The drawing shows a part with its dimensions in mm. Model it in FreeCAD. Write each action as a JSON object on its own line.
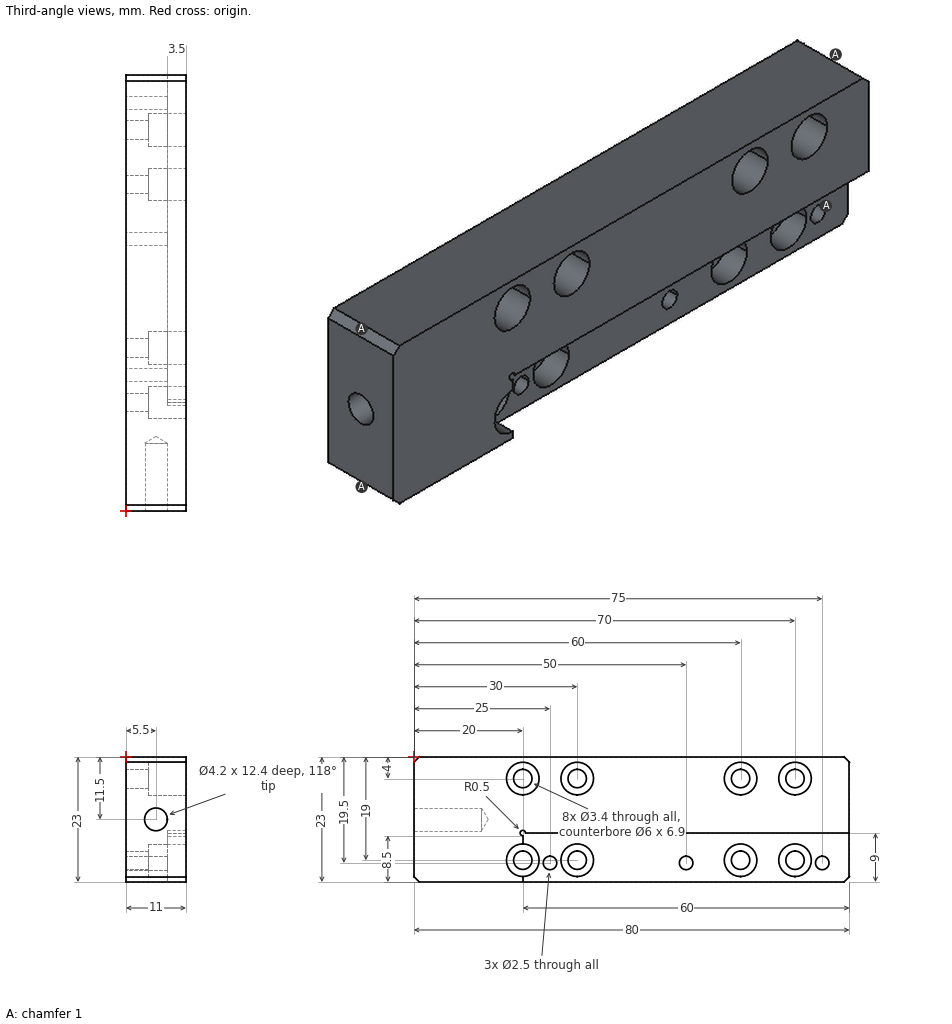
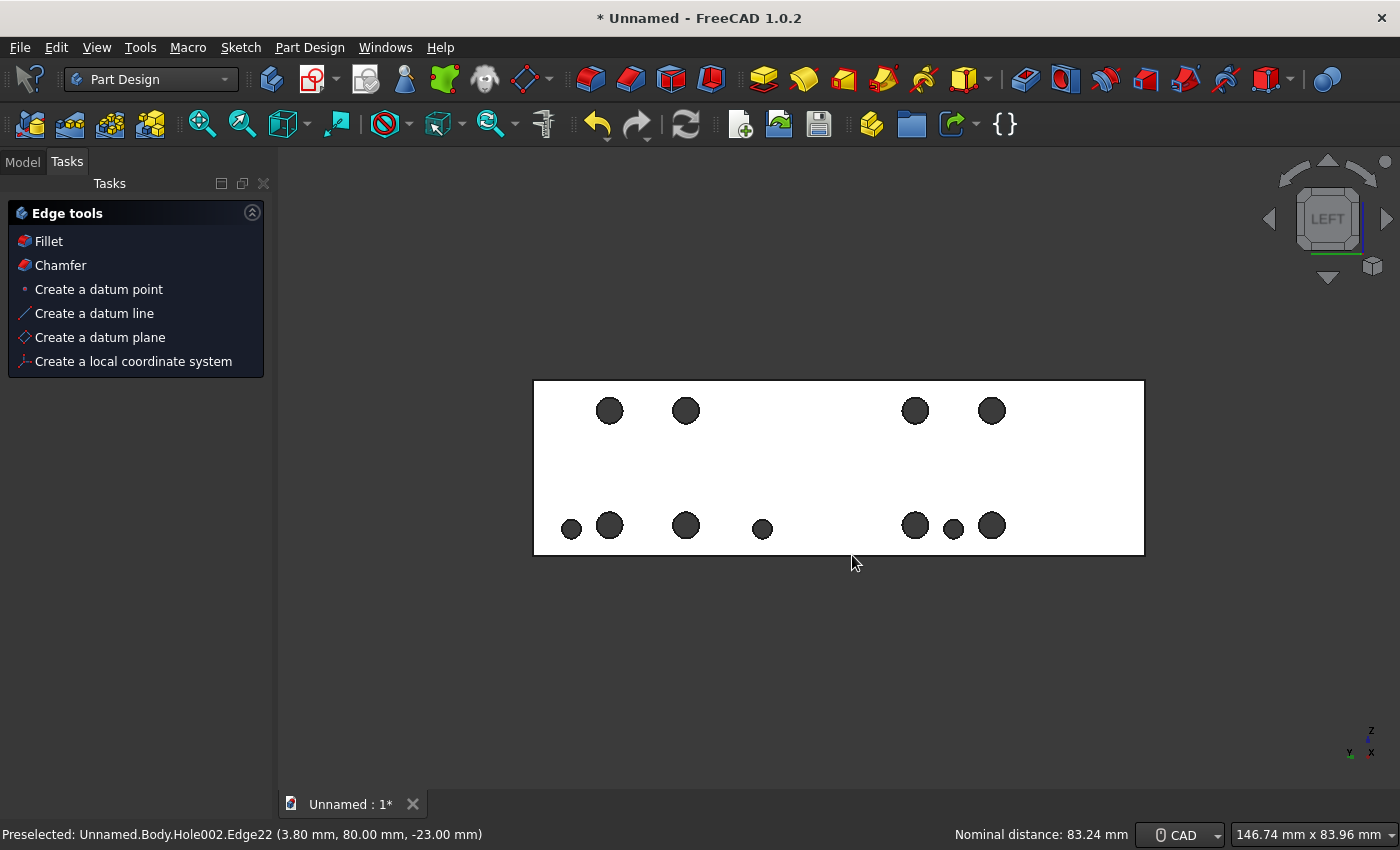
{"action": "key", "text": "v 3"}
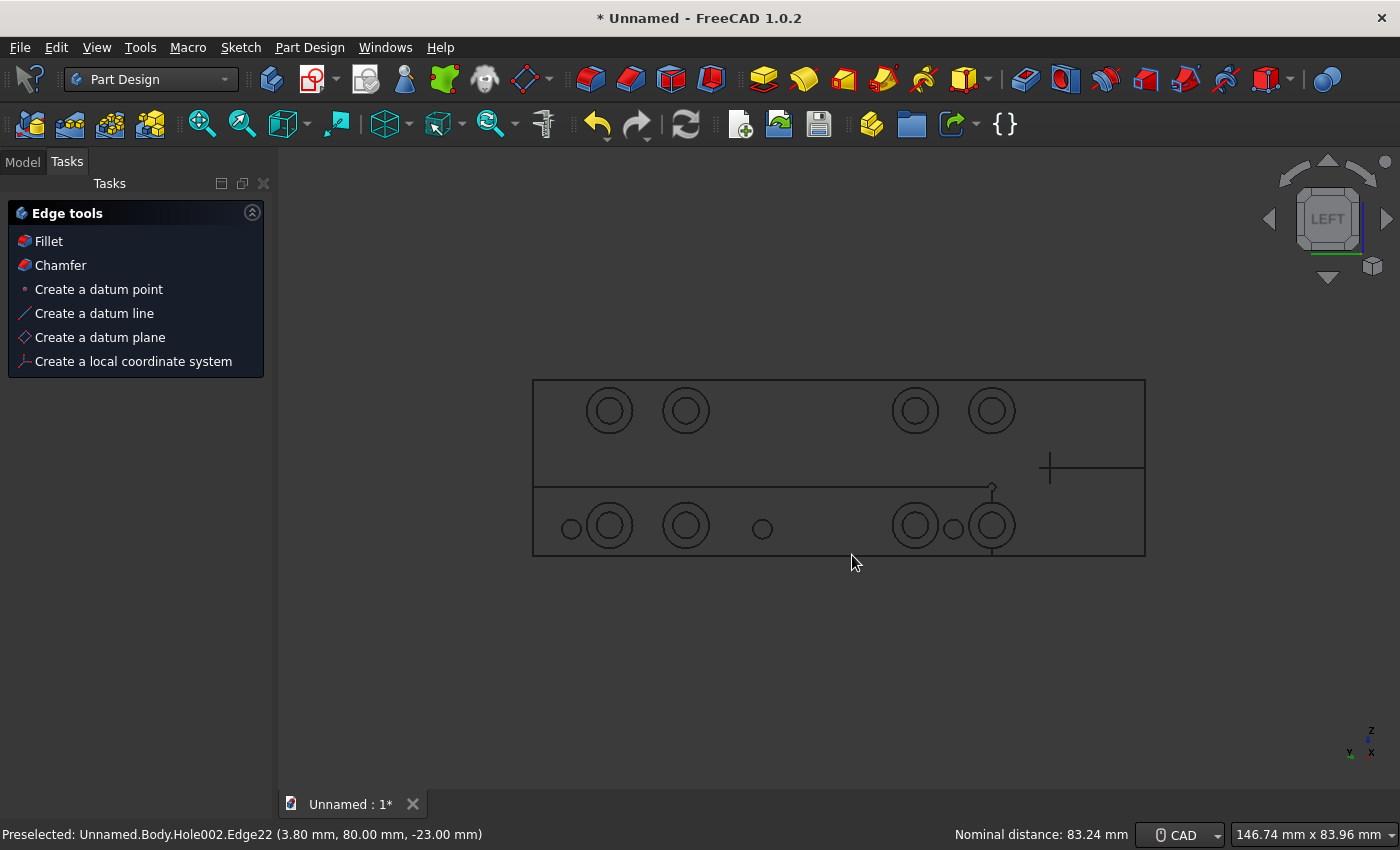
{"action": "key", "text": "0"}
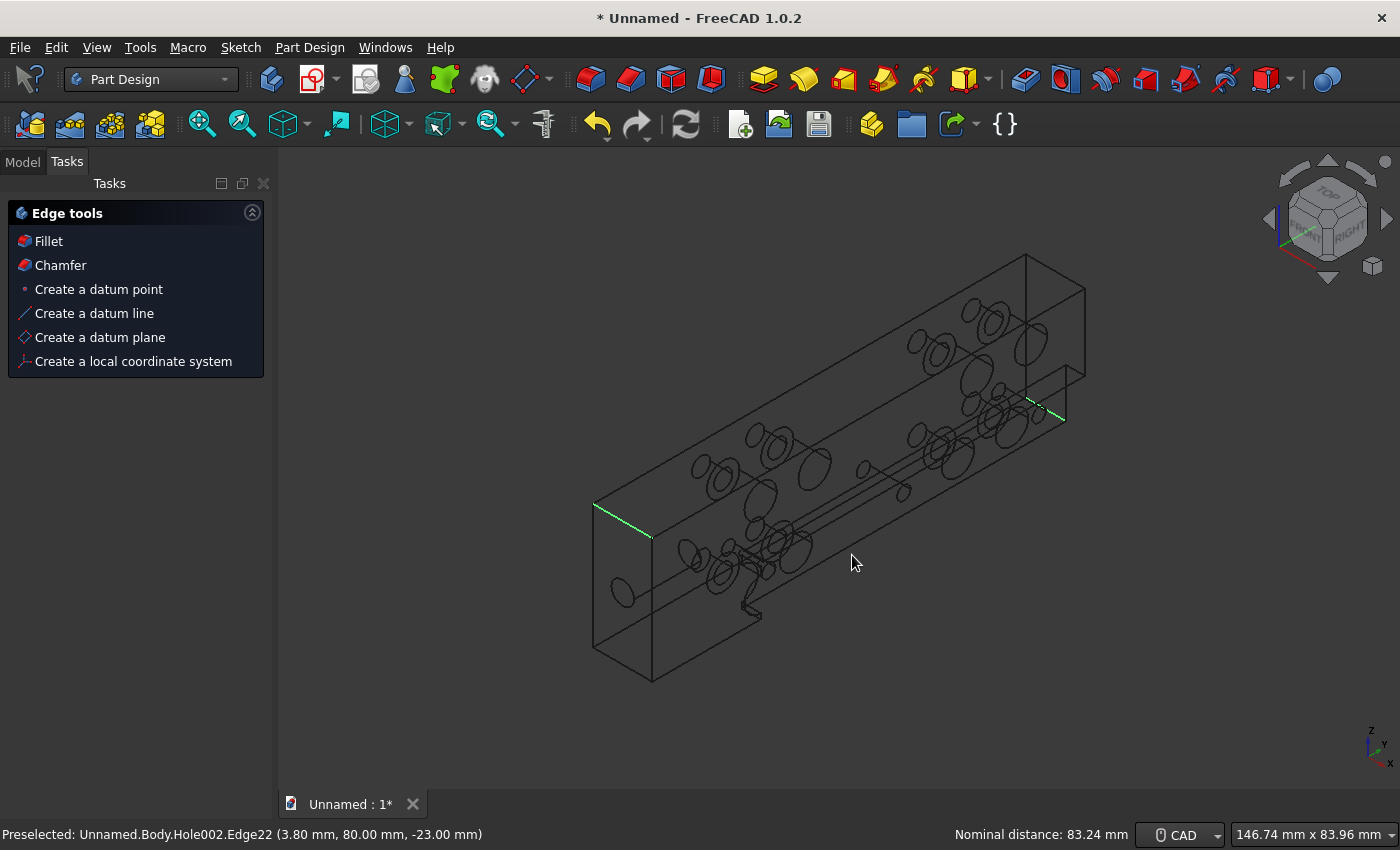
{"action": "left_click", "coordinate": [1055, 270], "text": "ctrl"}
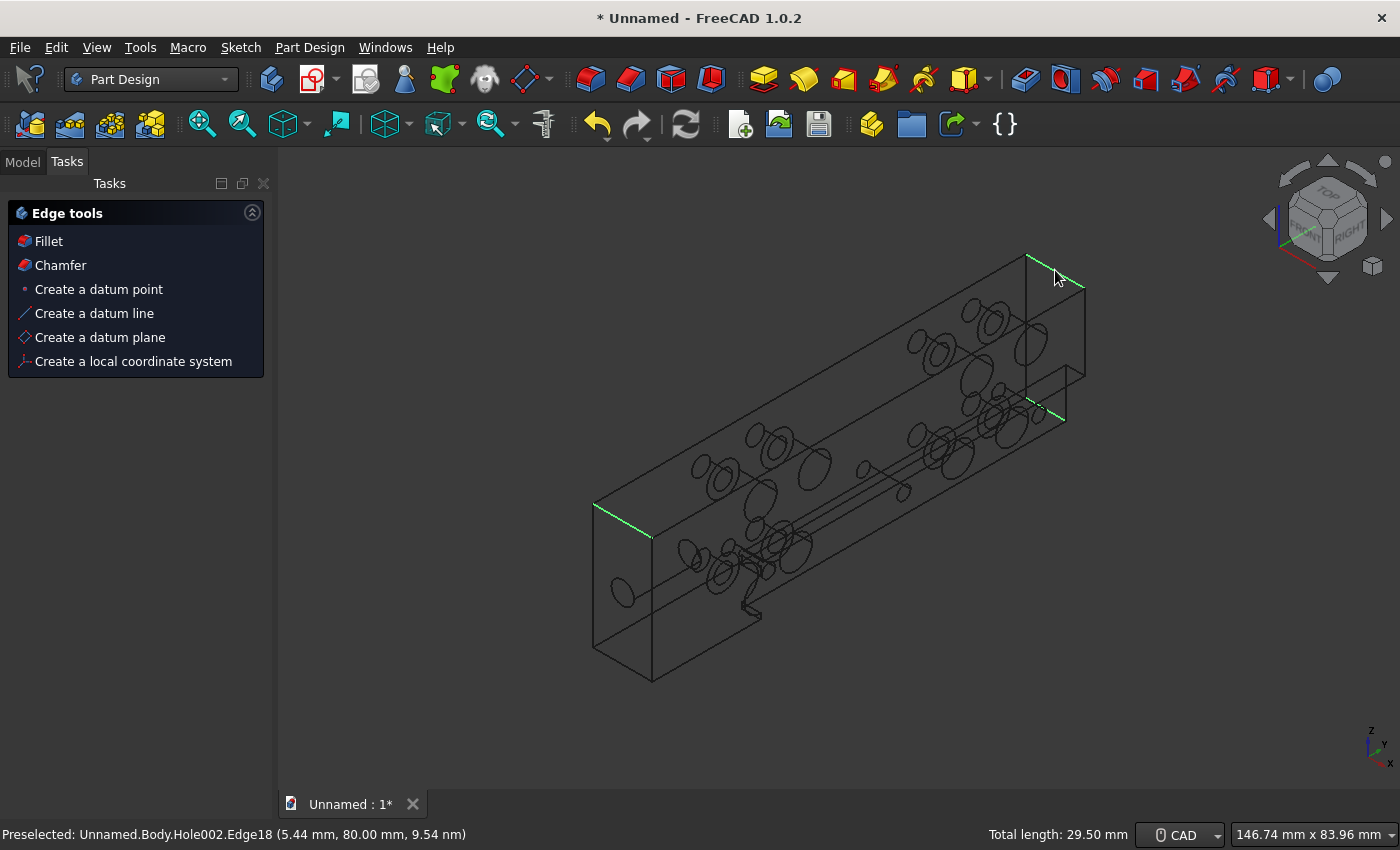
{"action": "left_click", "coordinate": [623, 664], "text": "ctrl"}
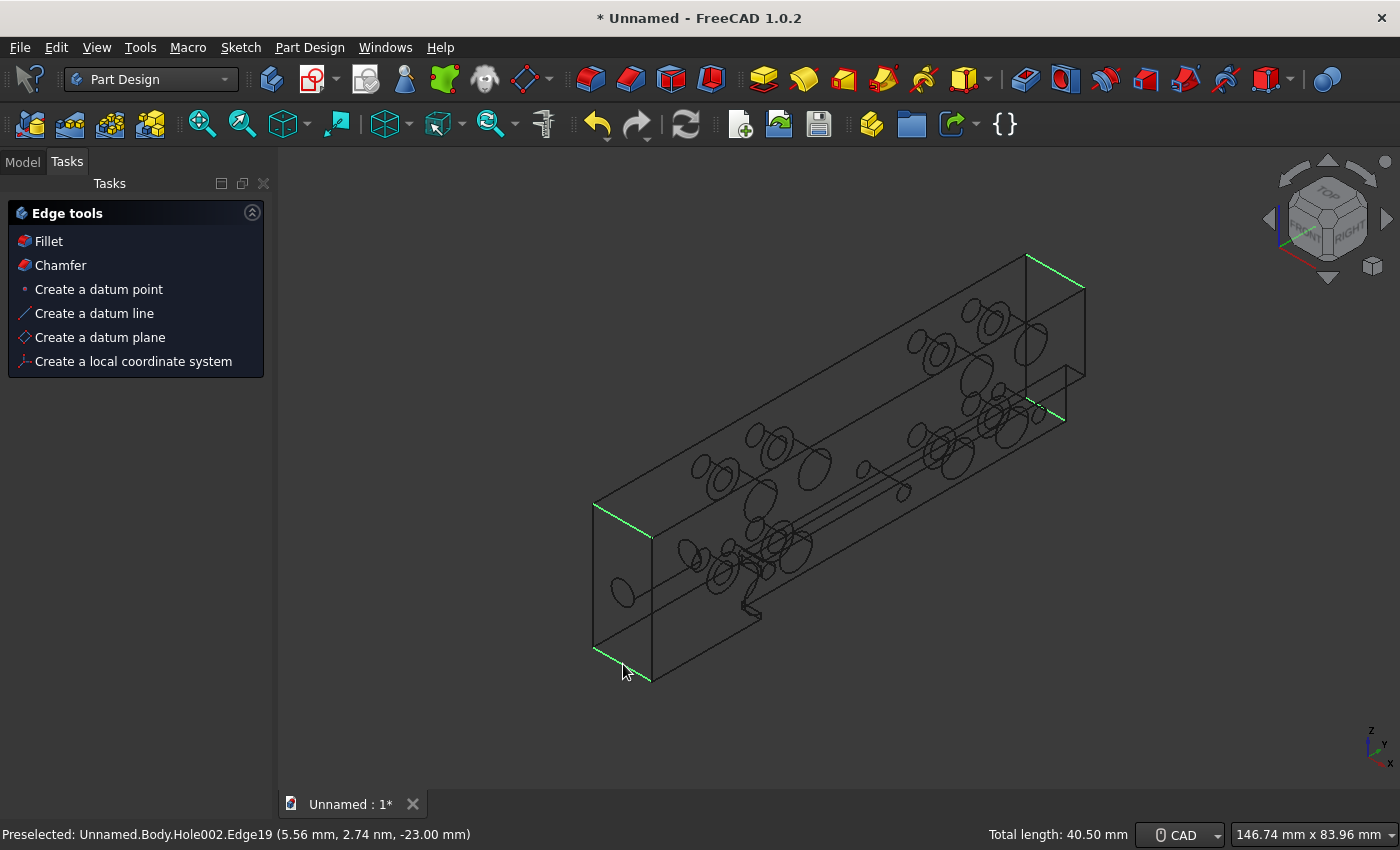
{"action": "key", "text": "v 1"}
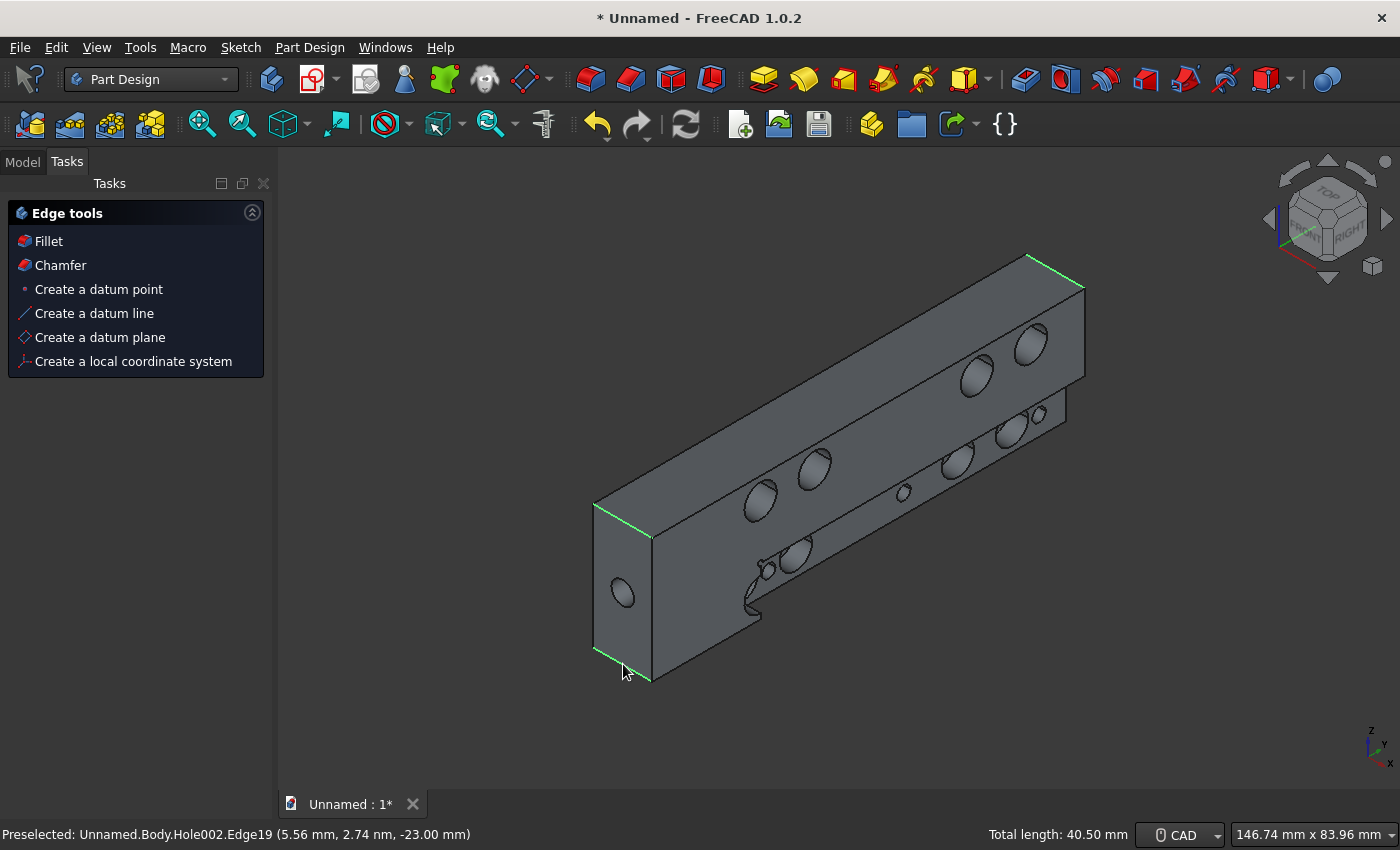
{"action": "left_click", "coordinate": [632, 80]}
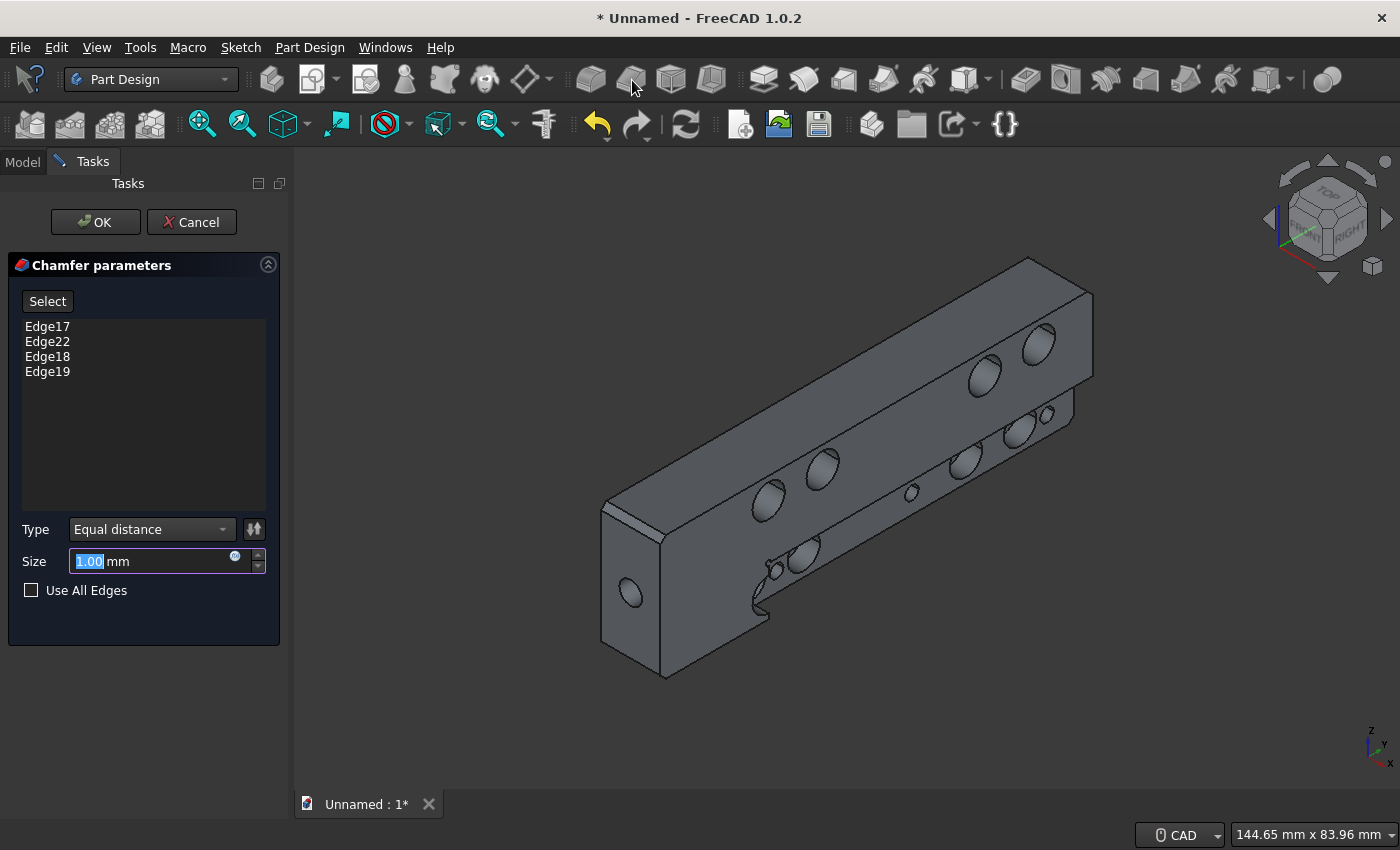
{"action": "type", "text": "1"}
{"action": "key", "text": "Tab"}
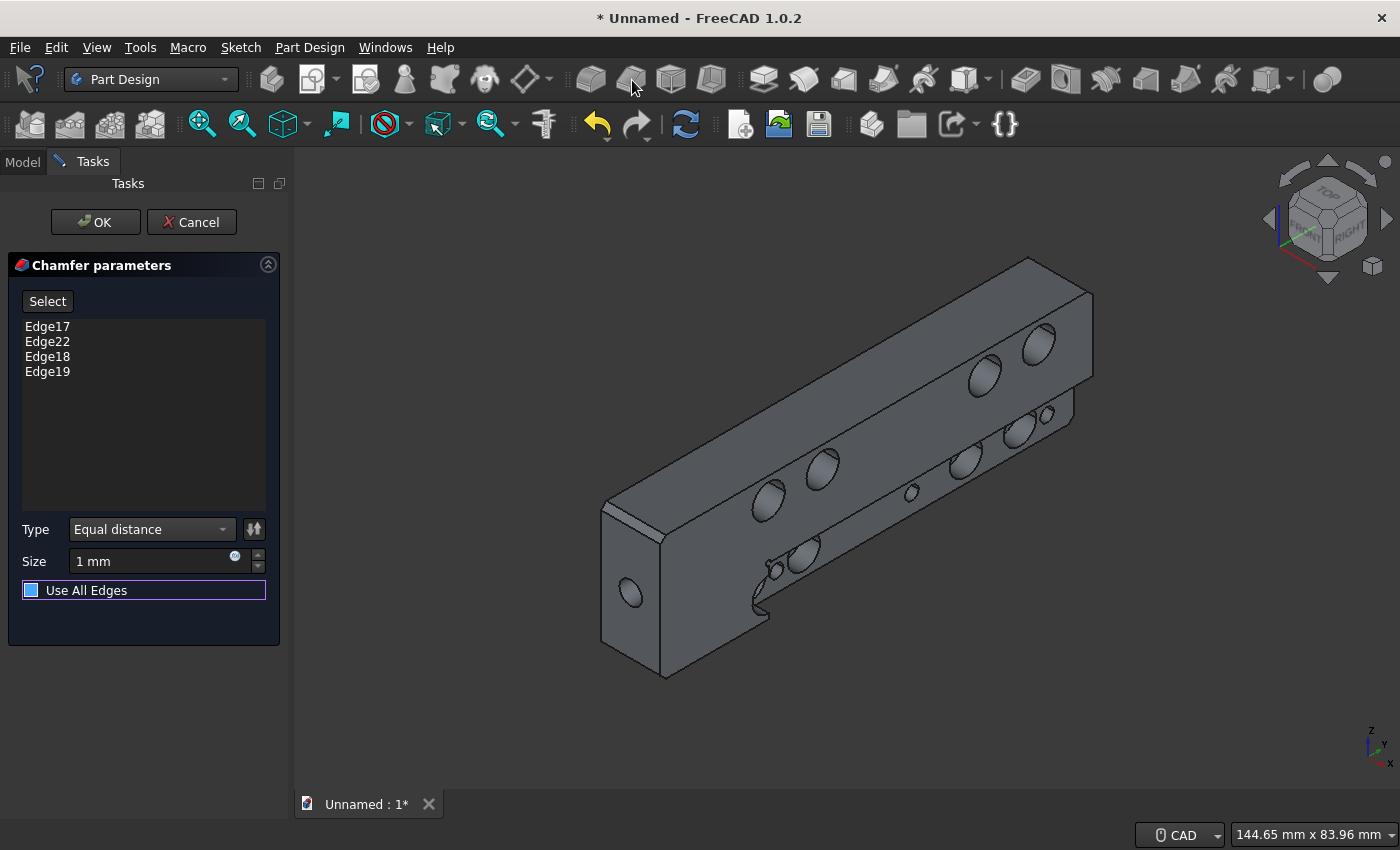
{"action": "left_click", "coordinate": [96, 222]}